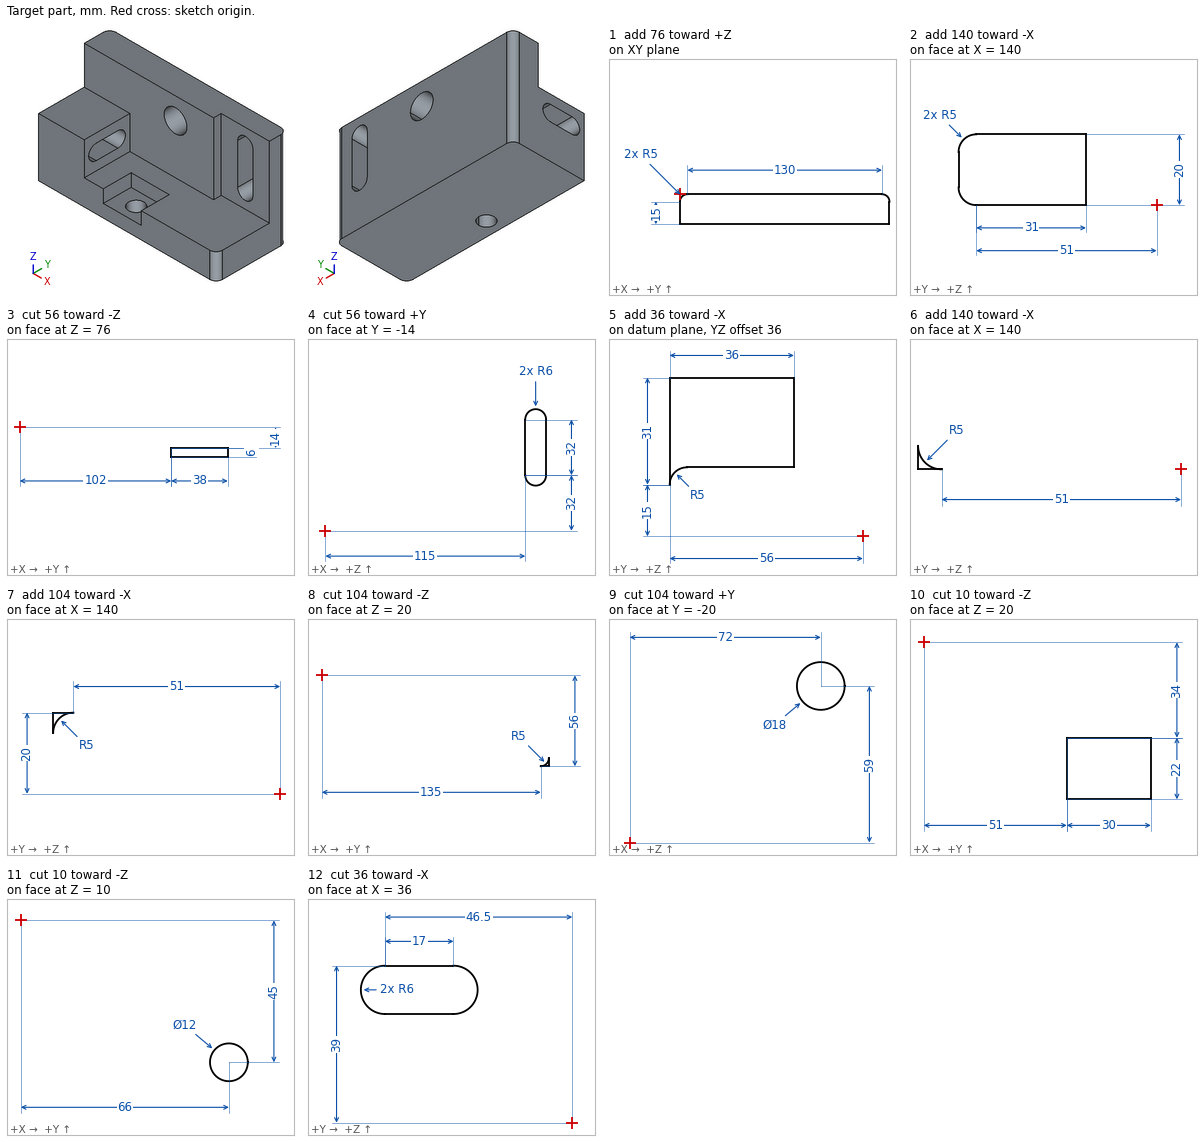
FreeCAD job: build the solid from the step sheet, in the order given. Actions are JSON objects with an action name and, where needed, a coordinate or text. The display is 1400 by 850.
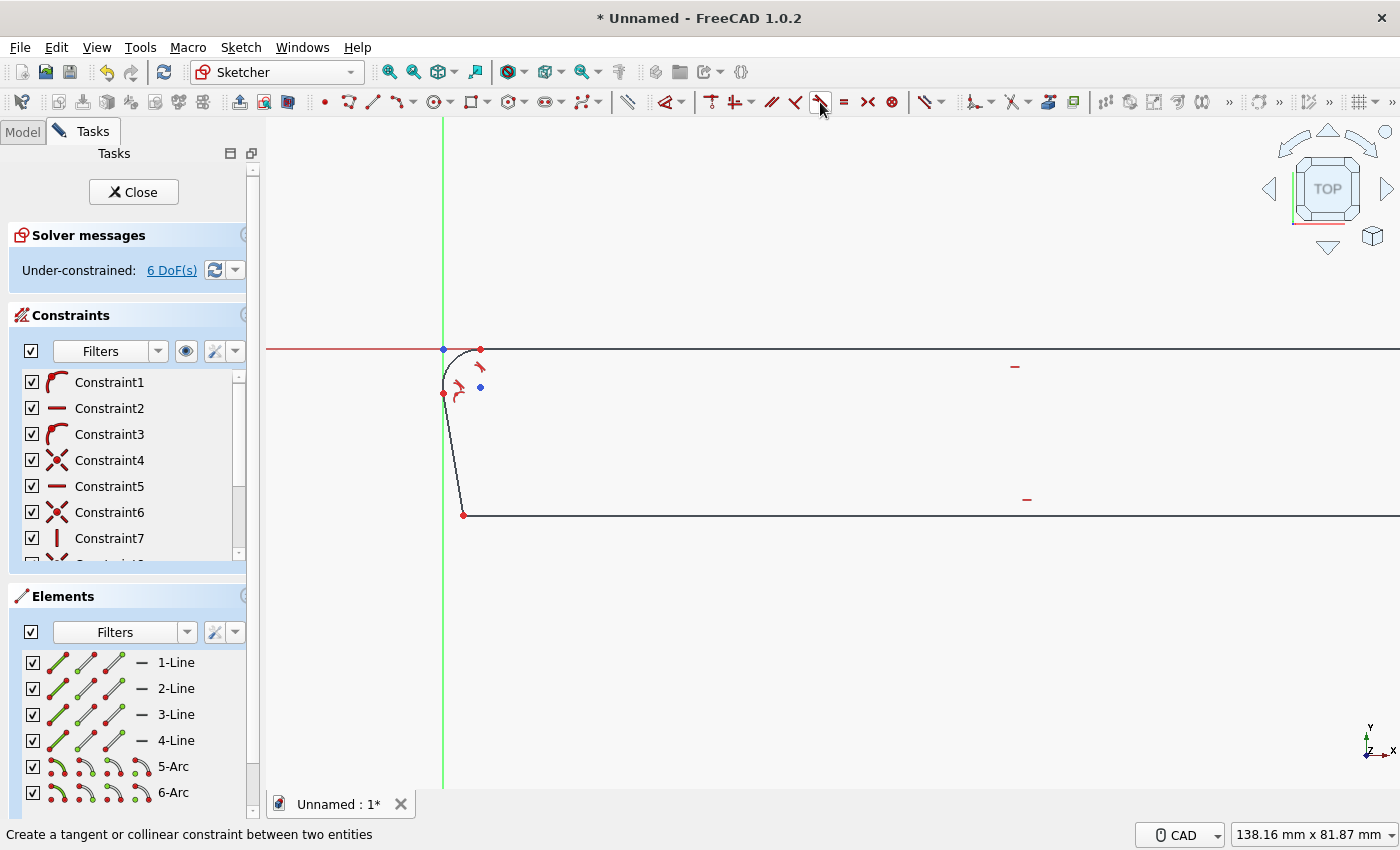
{"action": "scroll", "coordinate": [457, 479], "scroll_direction": "down", "scroll_amount": 3}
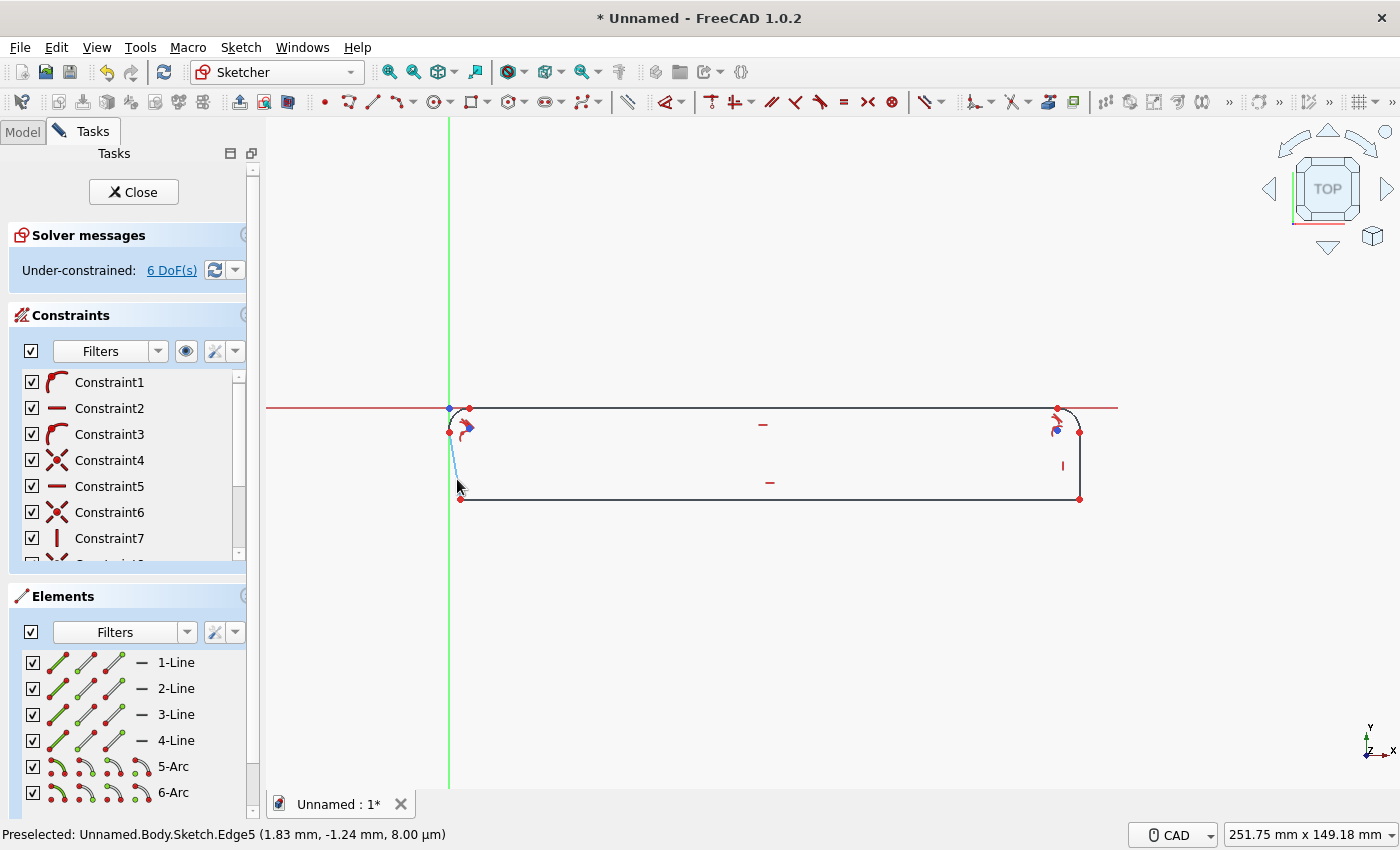
{"action": "left_click", "coordinate": [1080, 479]}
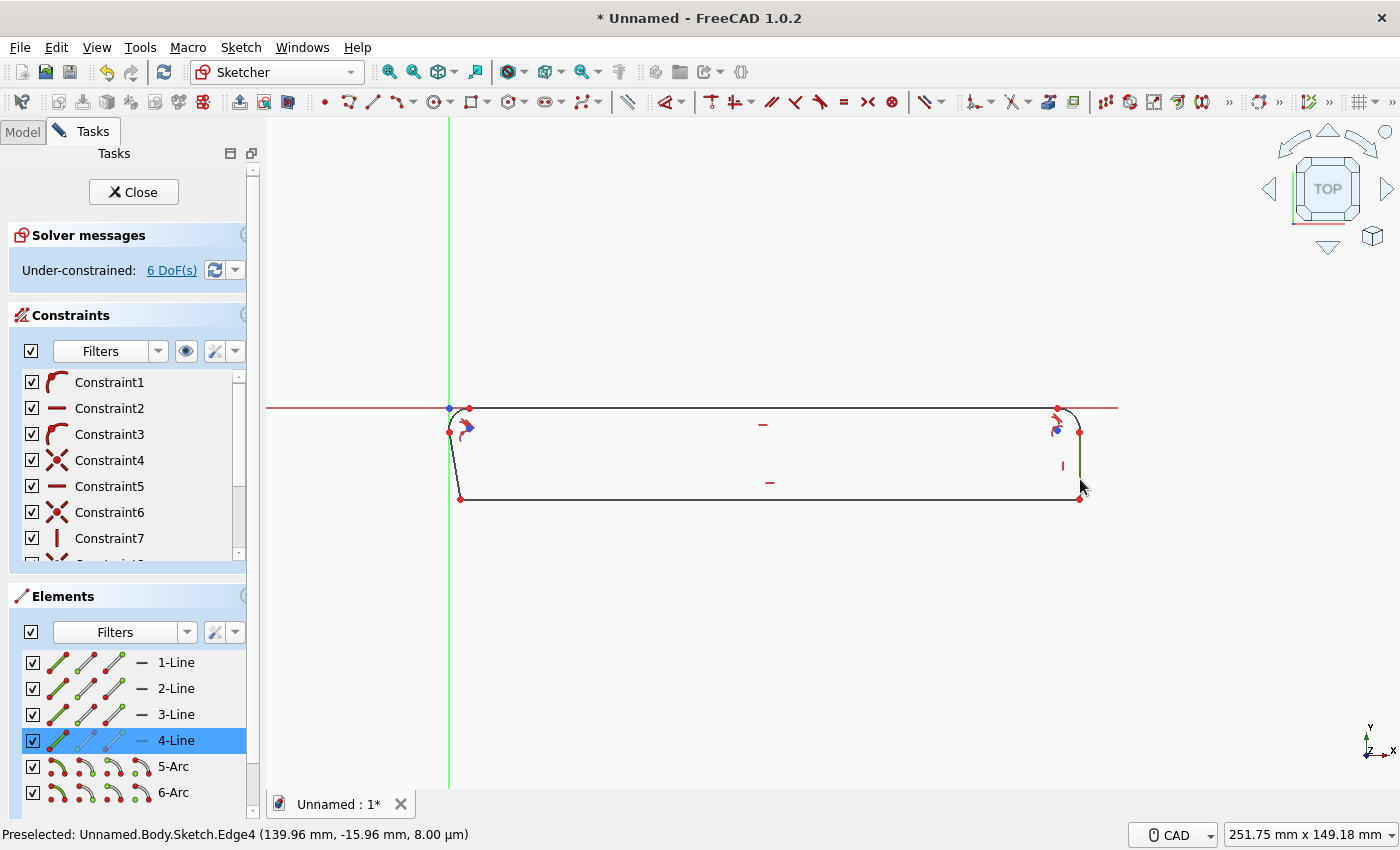
{"action": "scroll", "coordinate": [1078, 421], "scroll_direction": "up", "scroll_amount": 2}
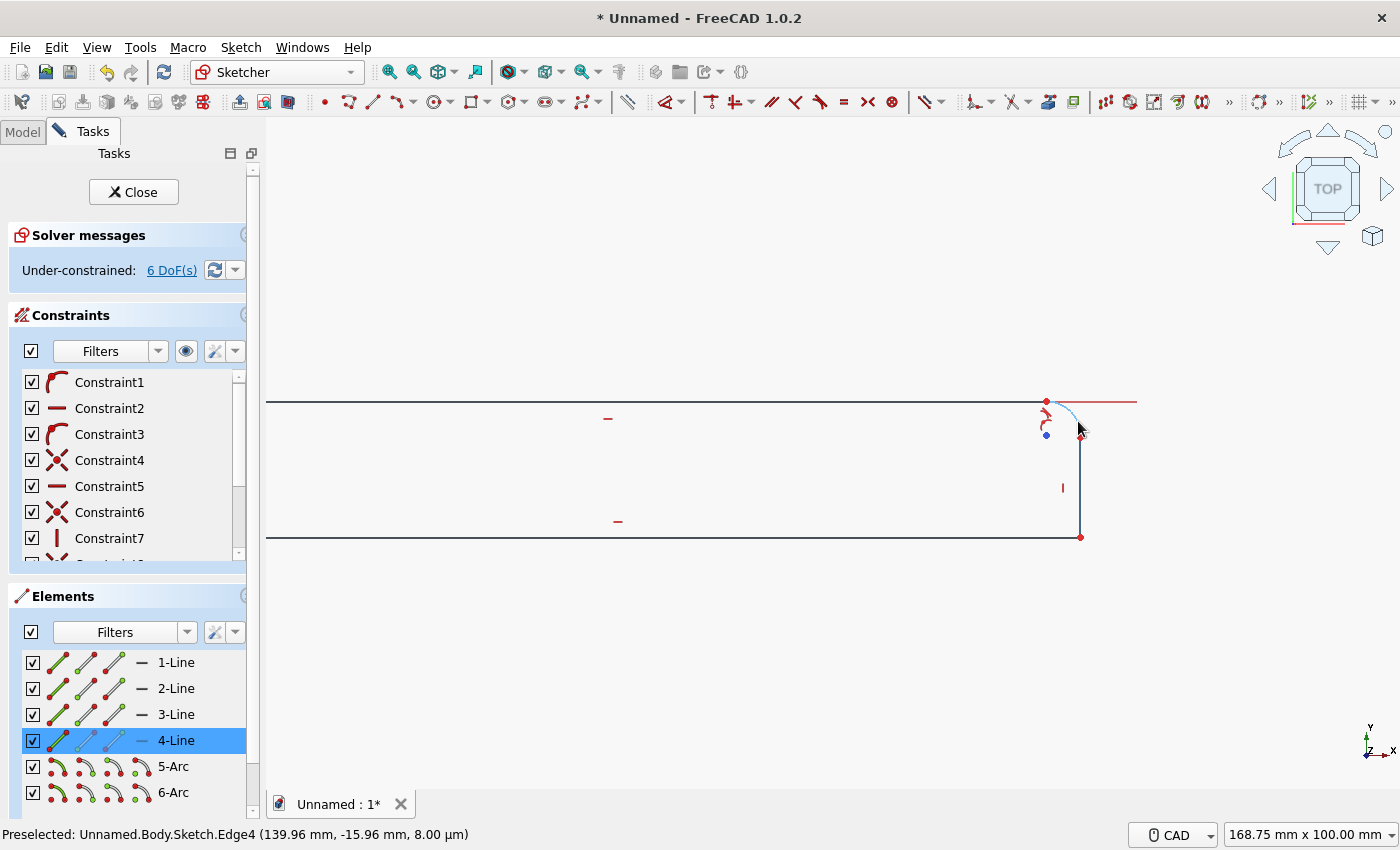
{"action": "left_click", "coordinate": [1078, 421]}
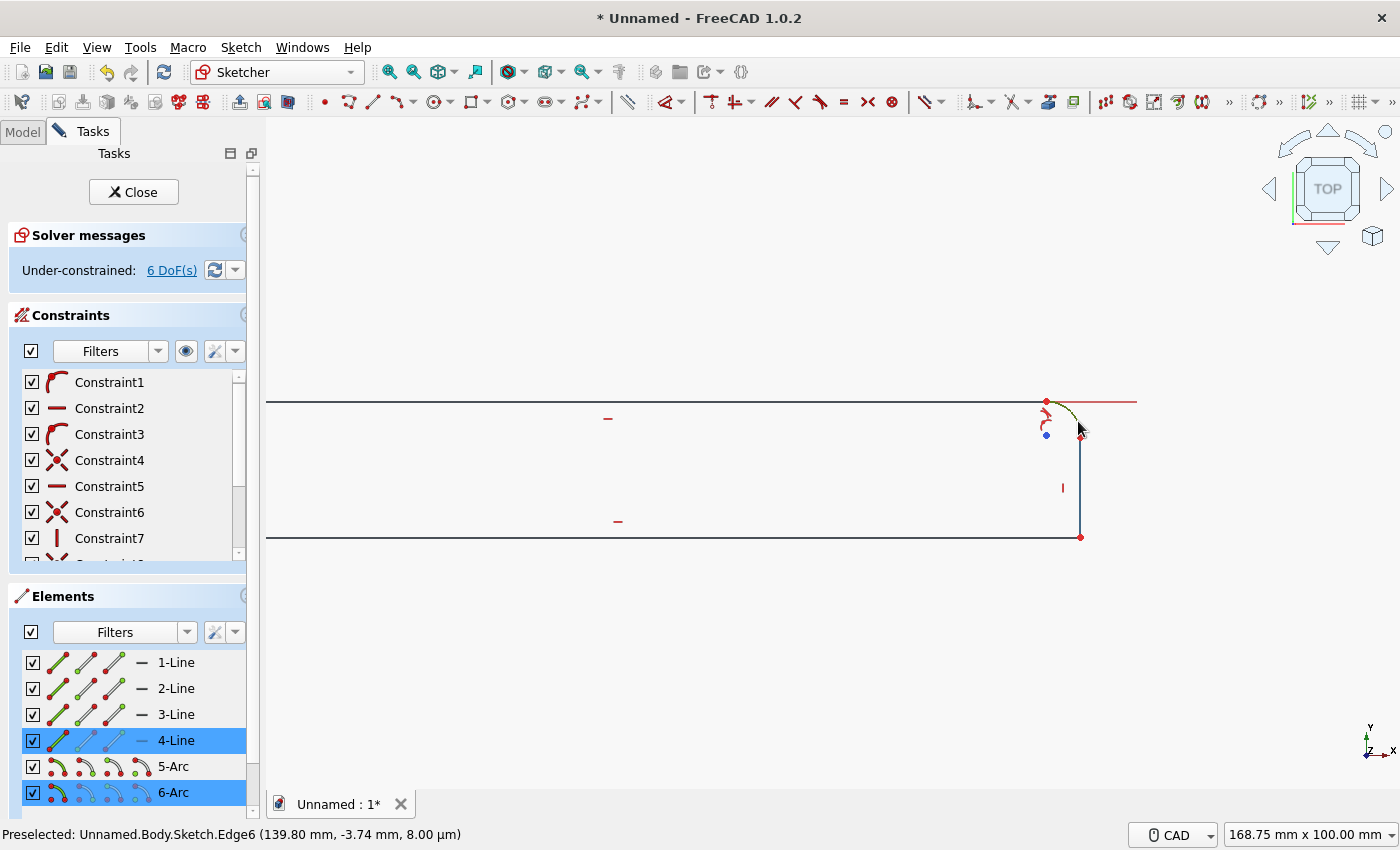
{"action": "left_click", "coordinate": [820, 102]}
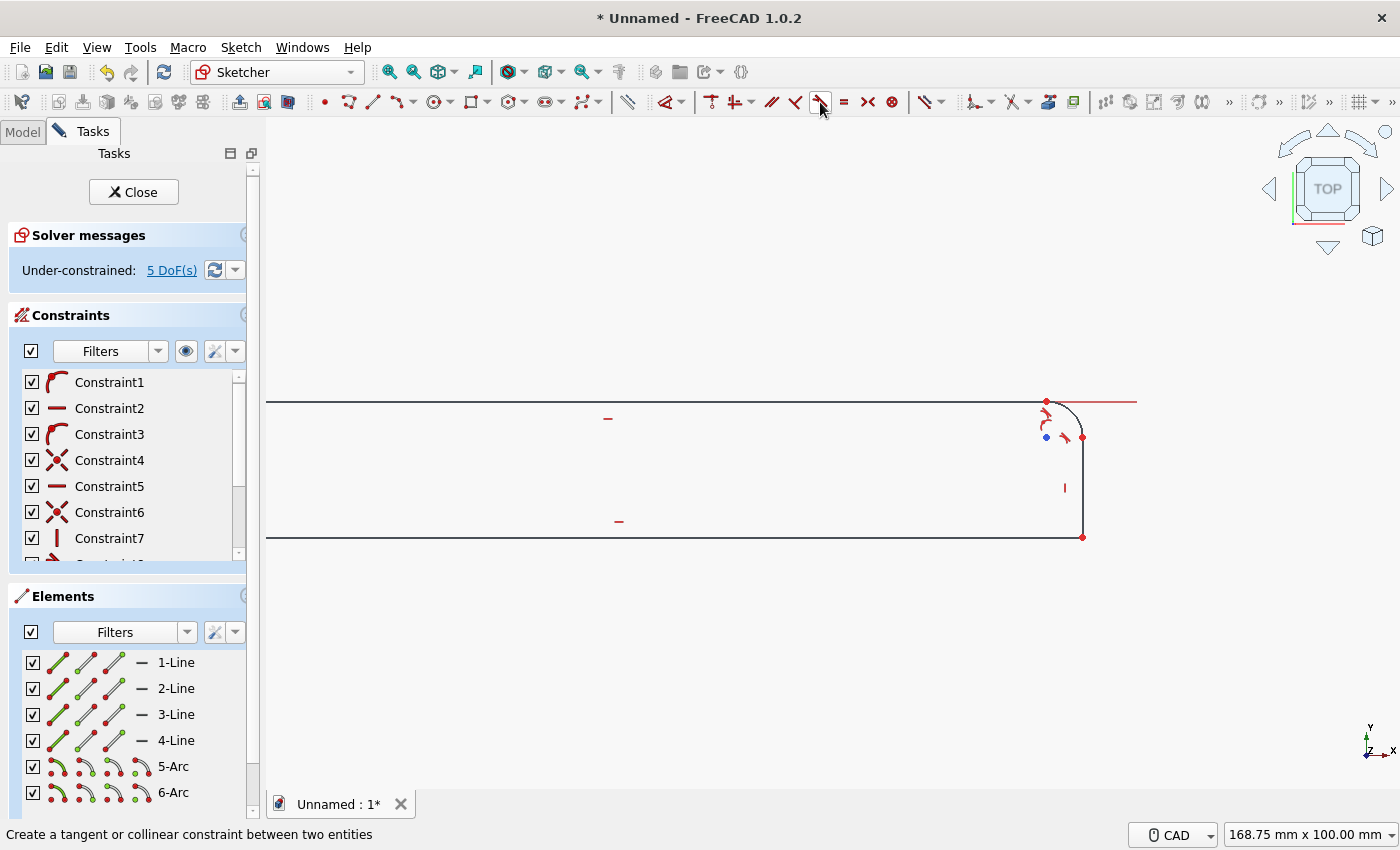
{"action": "scroll", "coordinate": [1078, 421], "scroll_direction": "down", "scroll_amount": 2}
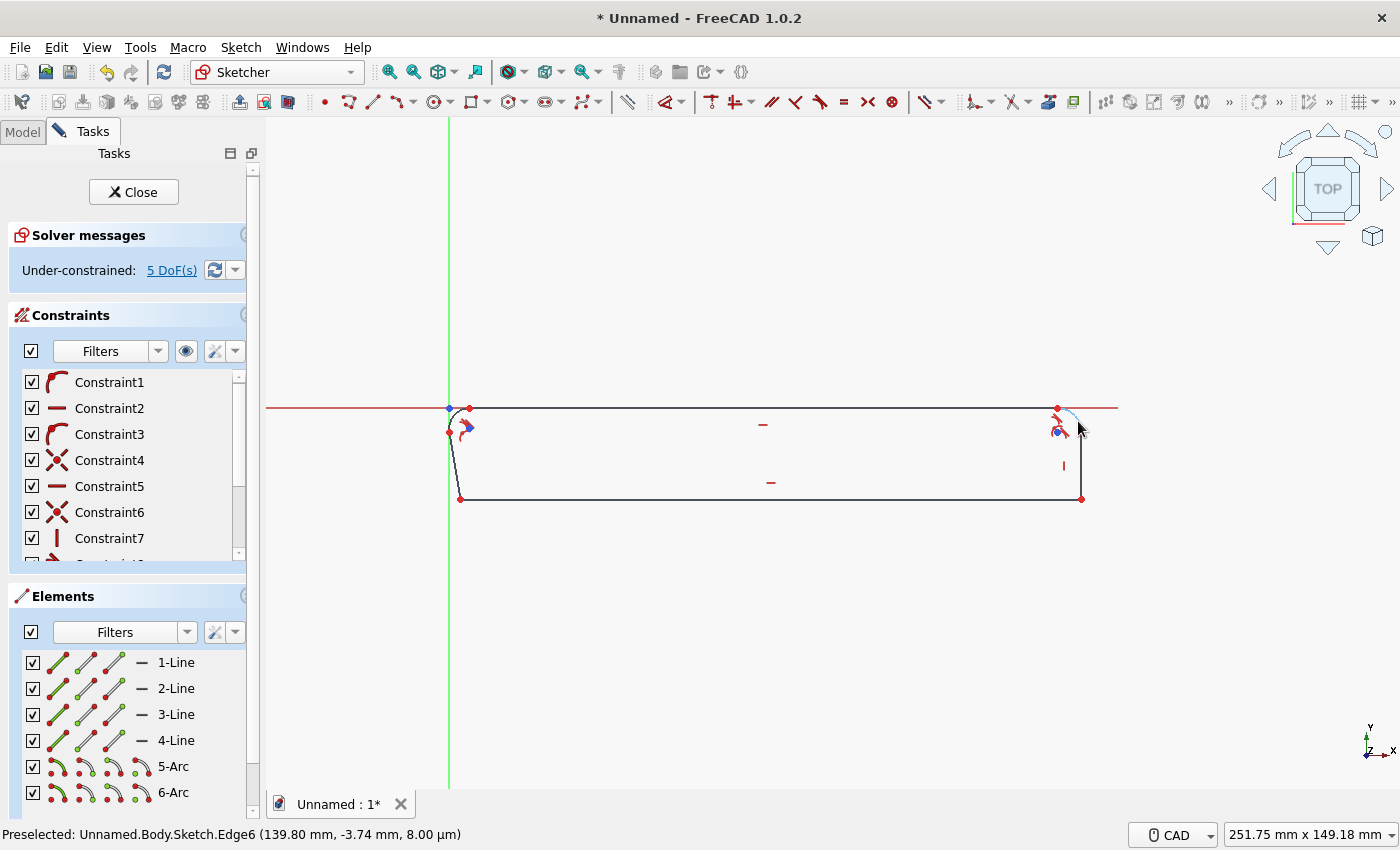
{"action": "scroll", "coordinate": [457, 479], "scroll_direction": "up", "scroll_amount": 3}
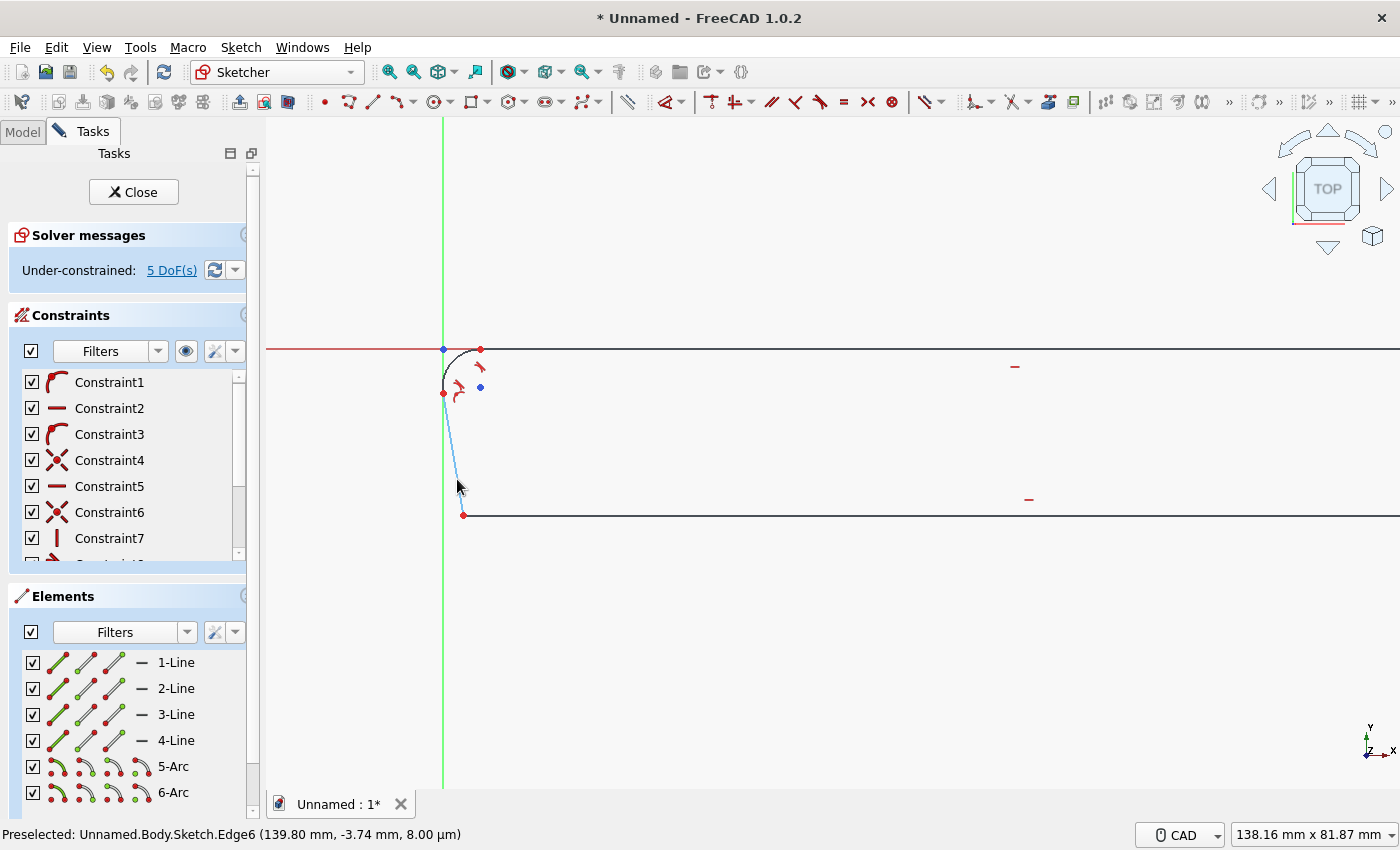
{"action": "left_click", "coordinate": [457, 479]}